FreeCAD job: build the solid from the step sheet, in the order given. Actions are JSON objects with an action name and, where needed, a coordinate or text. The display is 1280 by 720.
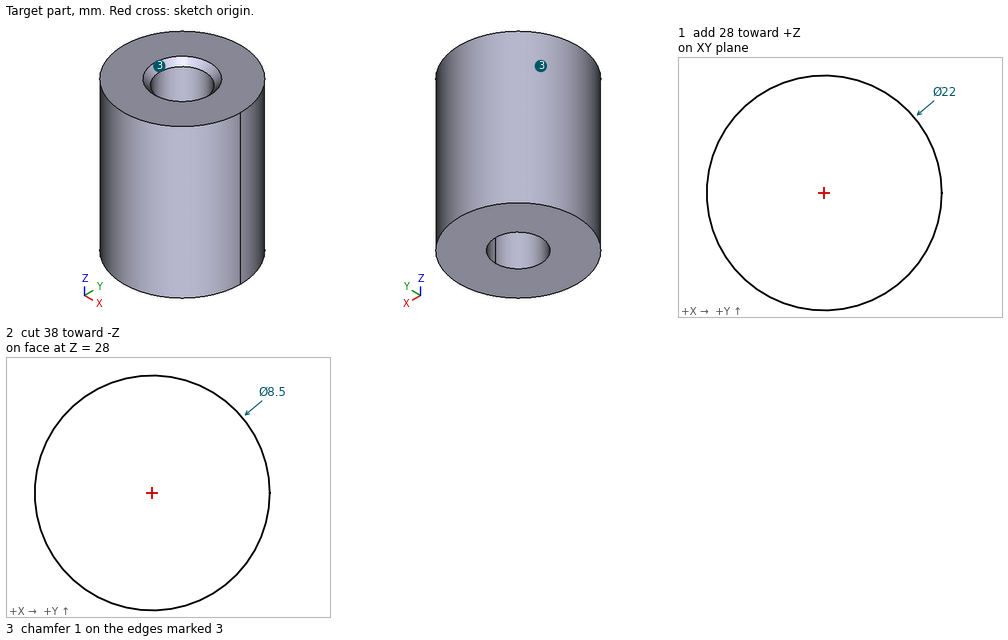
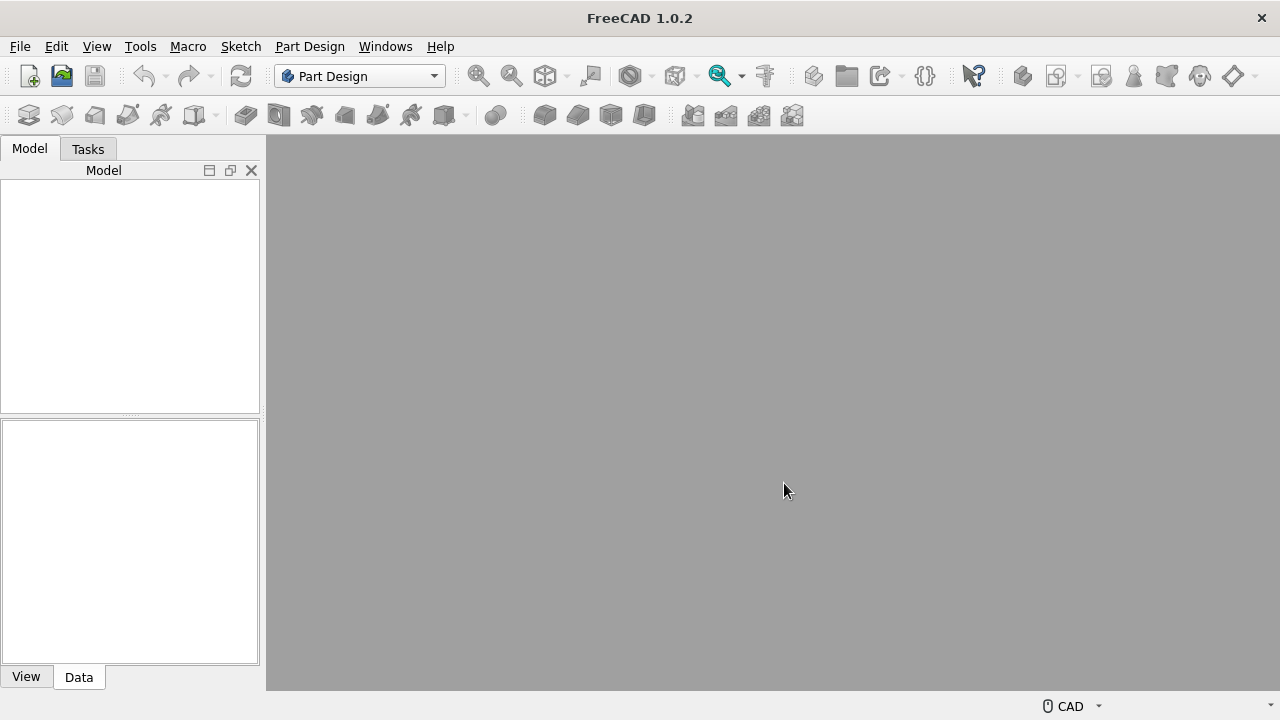
{"action": "left_click", "coordinate": [29, 76]}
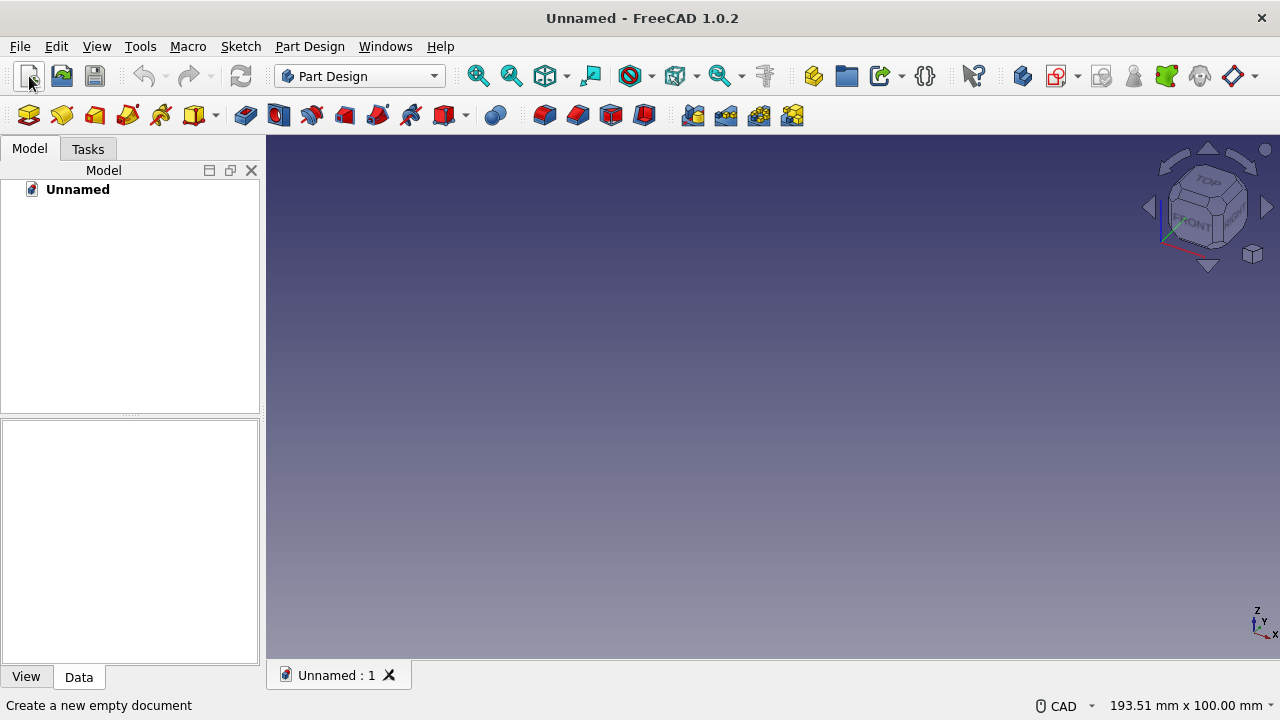
{"action": "left_click", "coordinate": [1056, 76]}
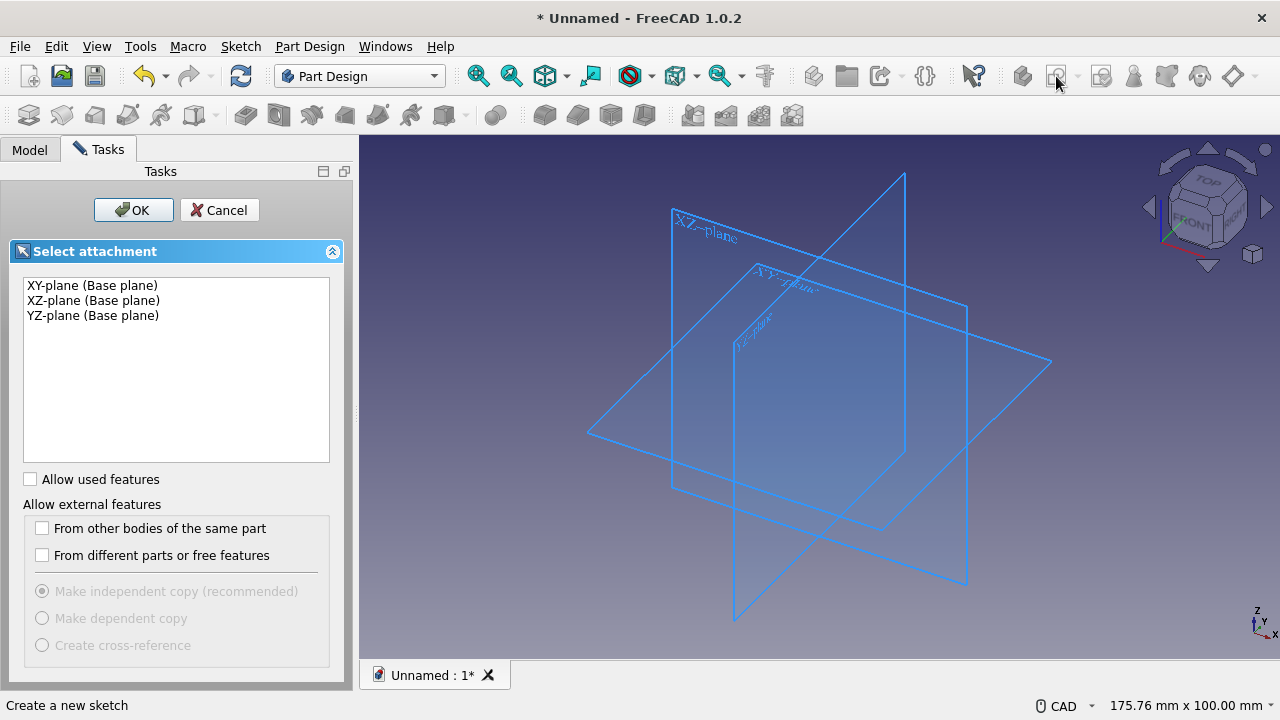
{"action": "left_click", "coordinate": [84, 286]}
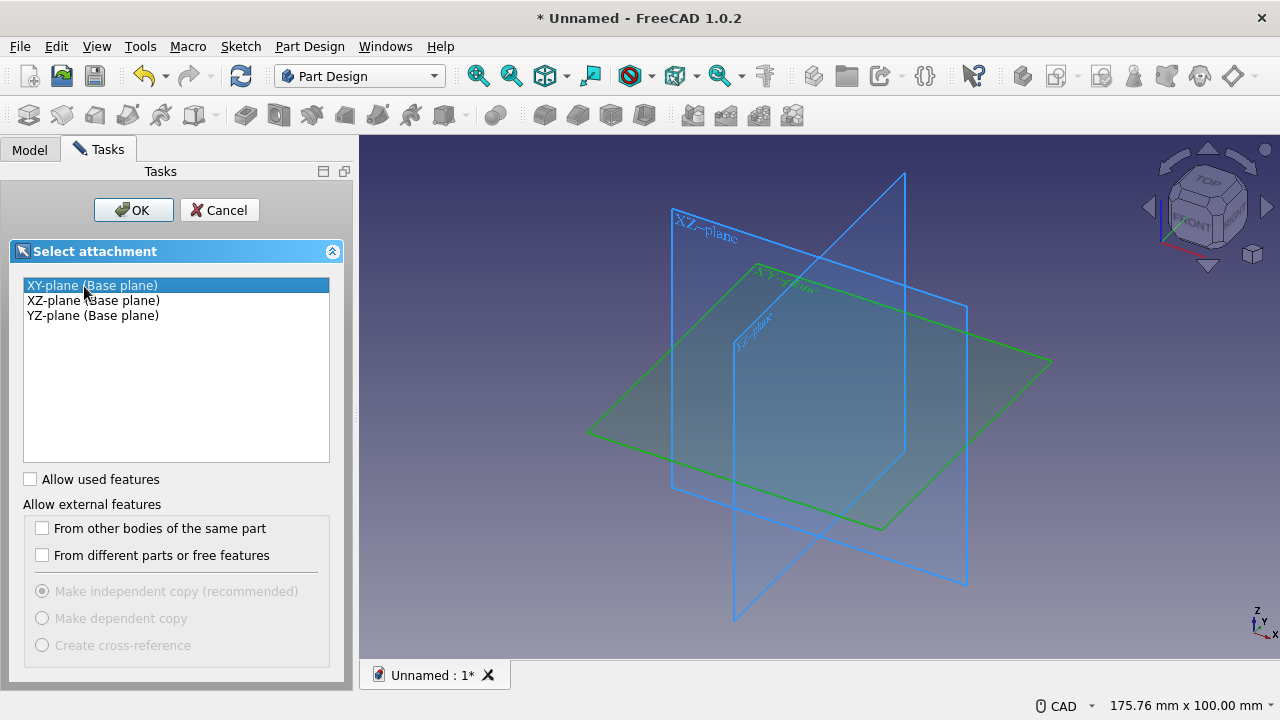
{"action": "left_click", "coordinate": [134, 210]}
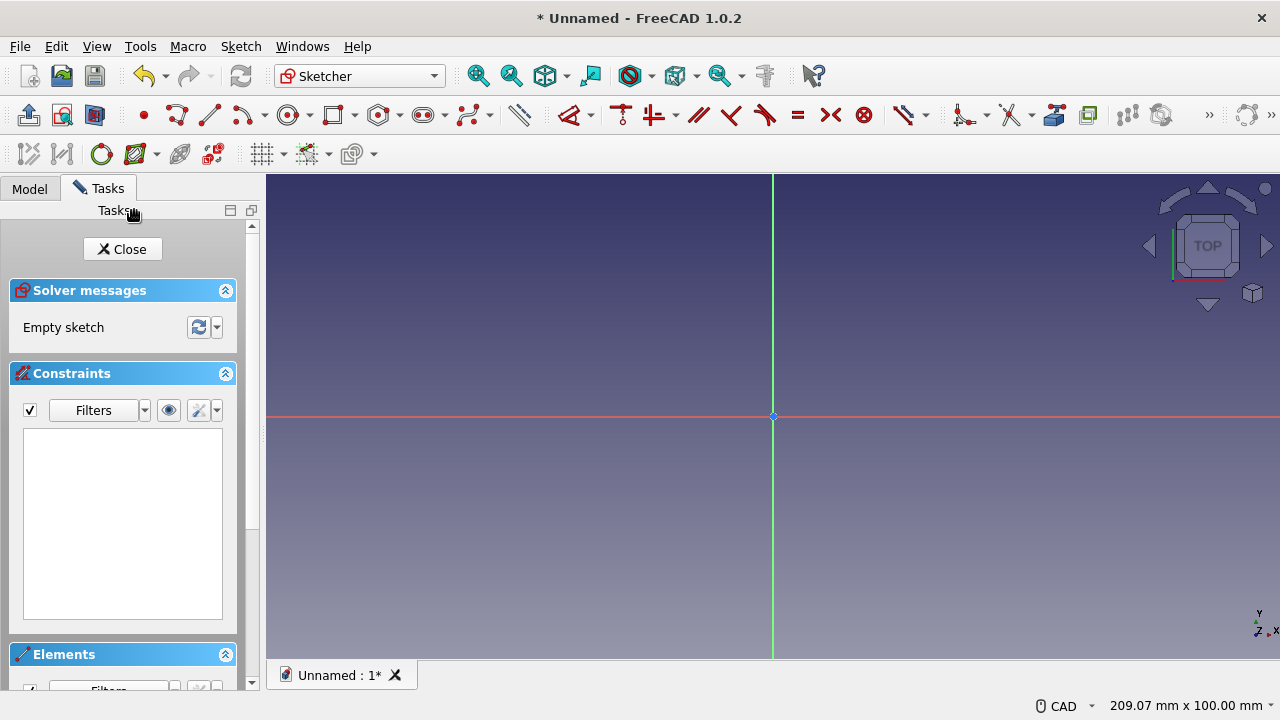
{"action": "scroll", "coordinate": [813, 416], "scroll_direction": "up", "scroll_amount": 5}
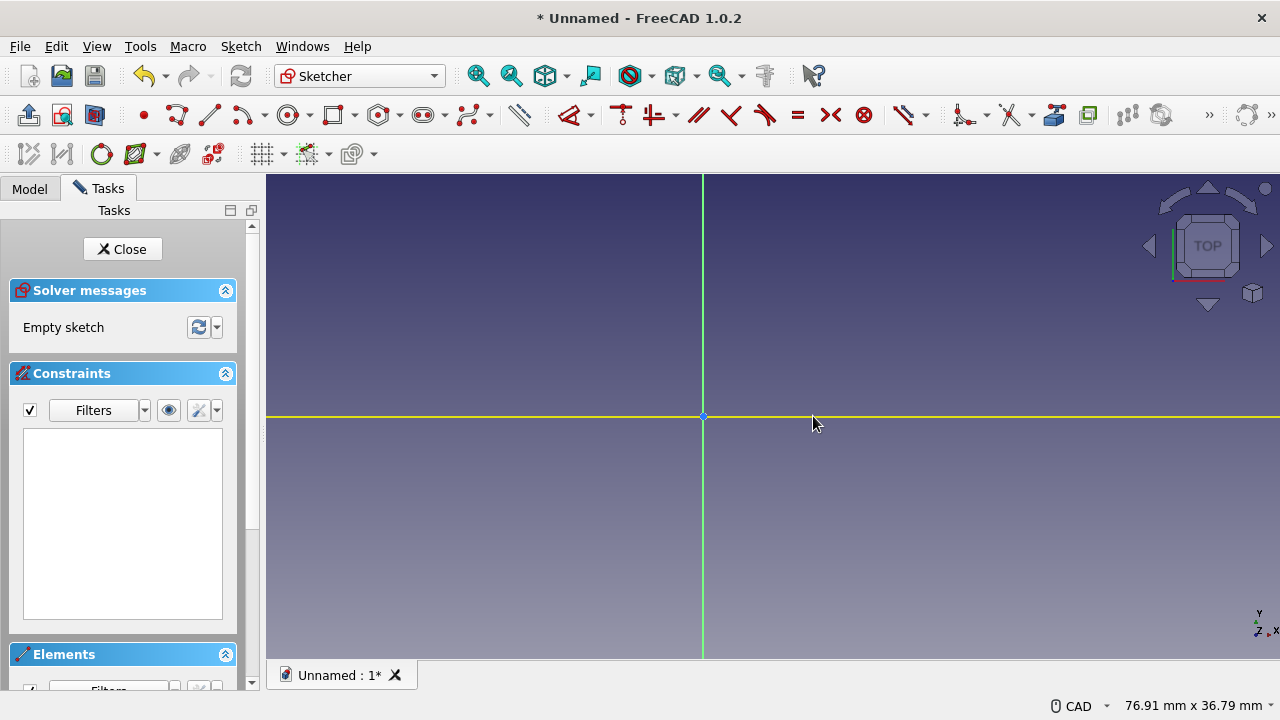
{"action": "left_click", "coordinate": [288, 116]}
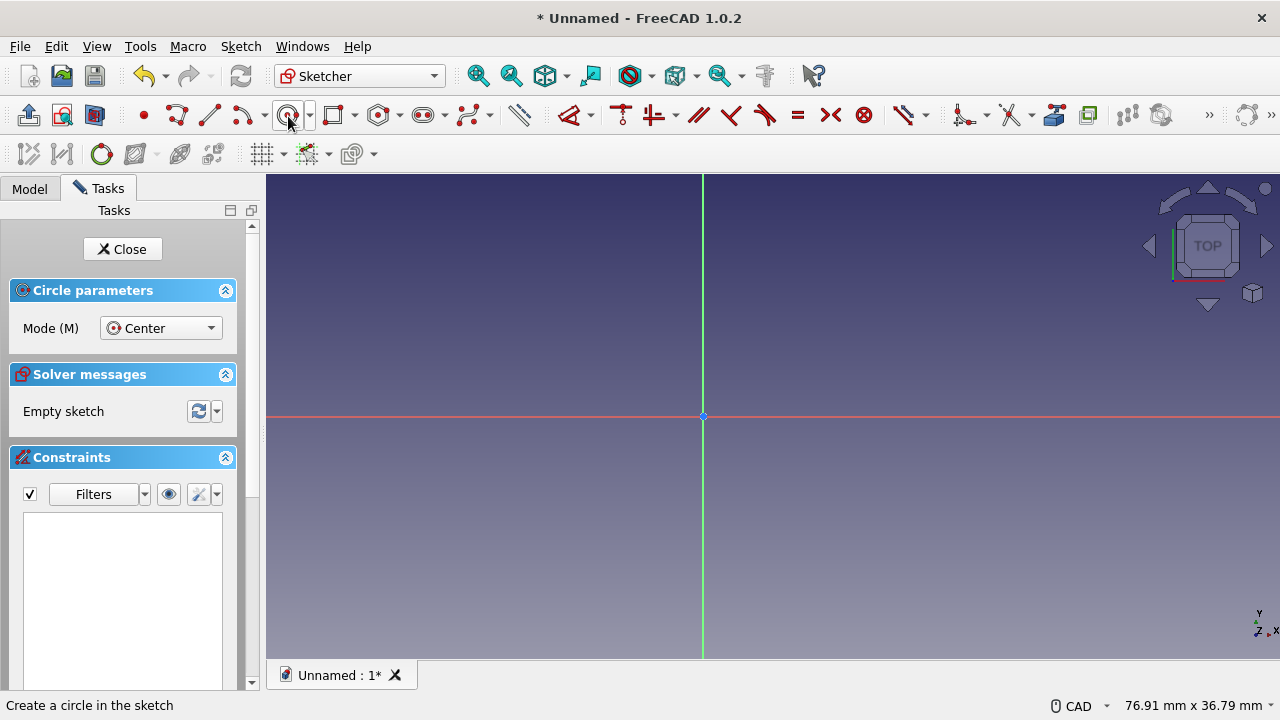
{"action": "left_click", "coordinate": [703, 416]}
{"action": "left_click", "coordinate": [806, 314]}
{"action": "key", "text": "Escape"}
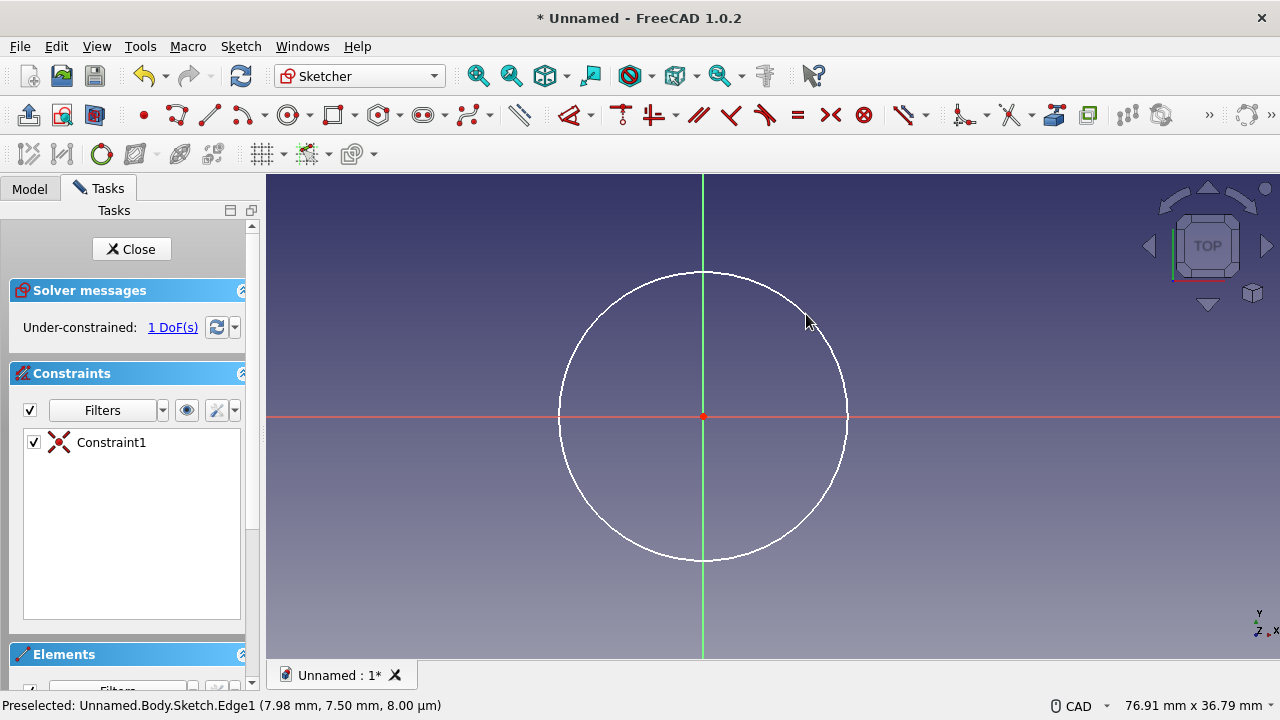
{"action": "left_click", "coordinate": [805, 314]}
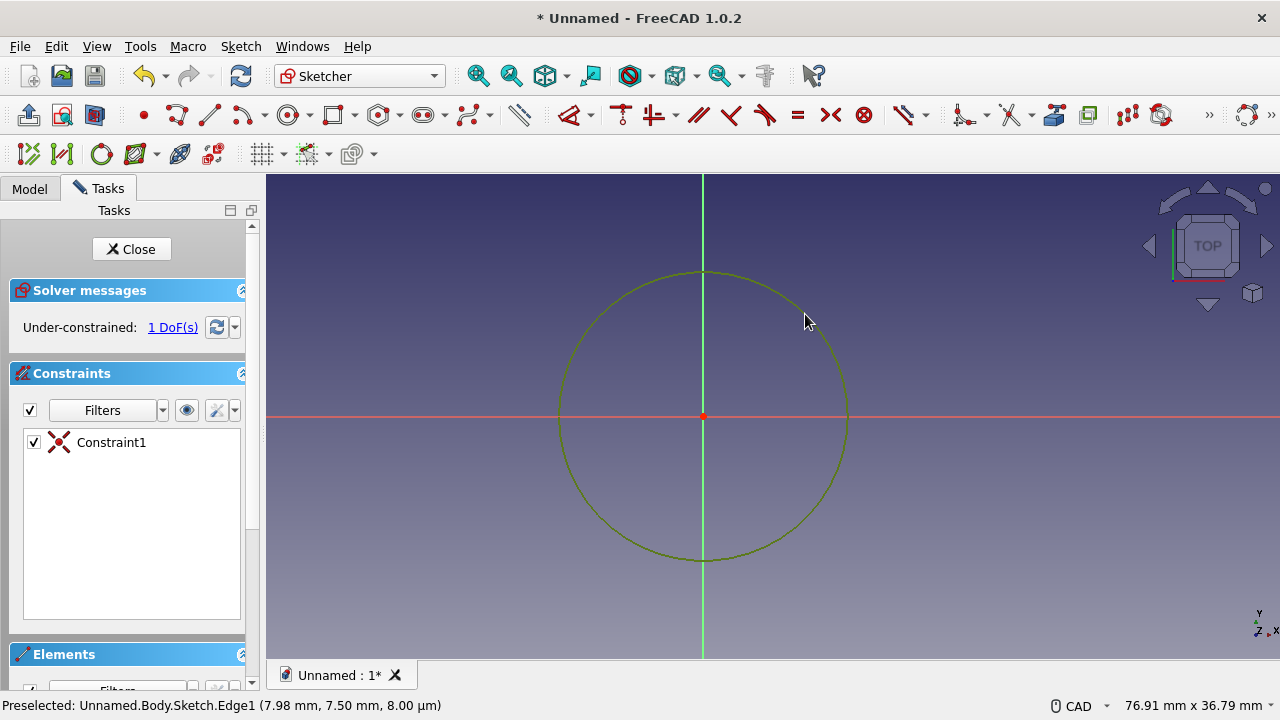
{"action": "left_click", "coordinate": [590, 116]}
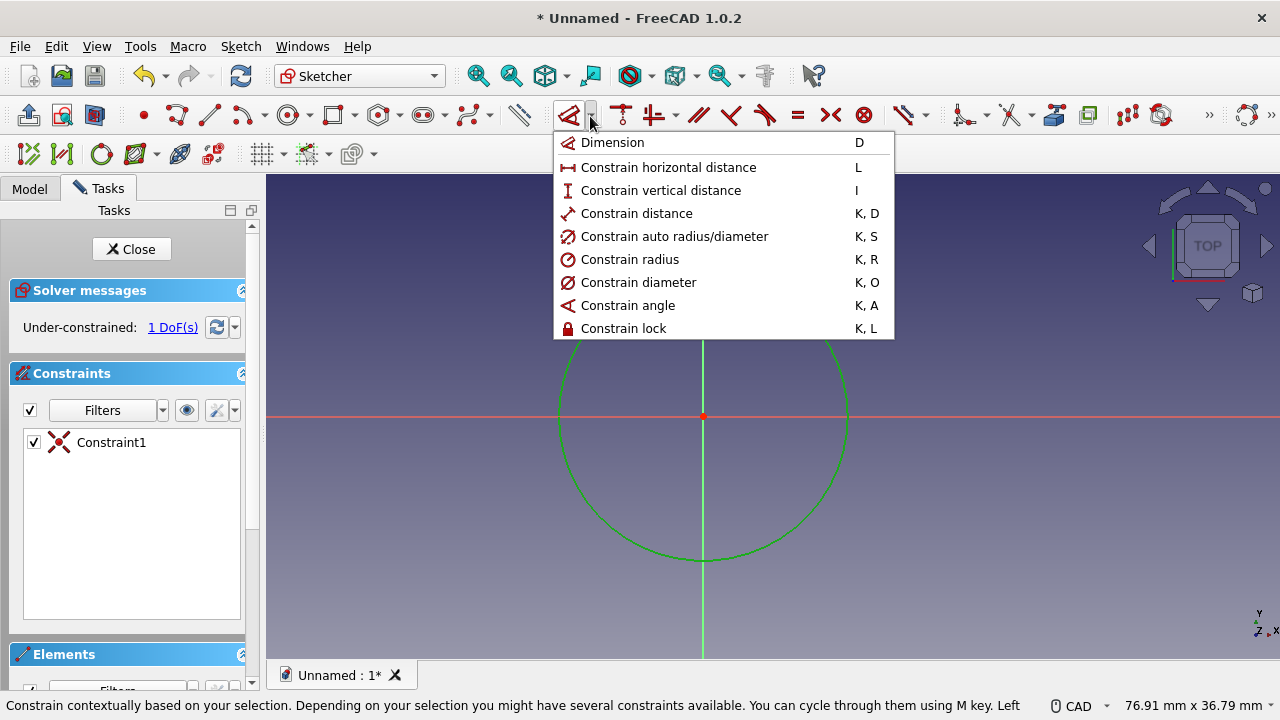
{"action": "left_click", "coordinate": [724, 282]}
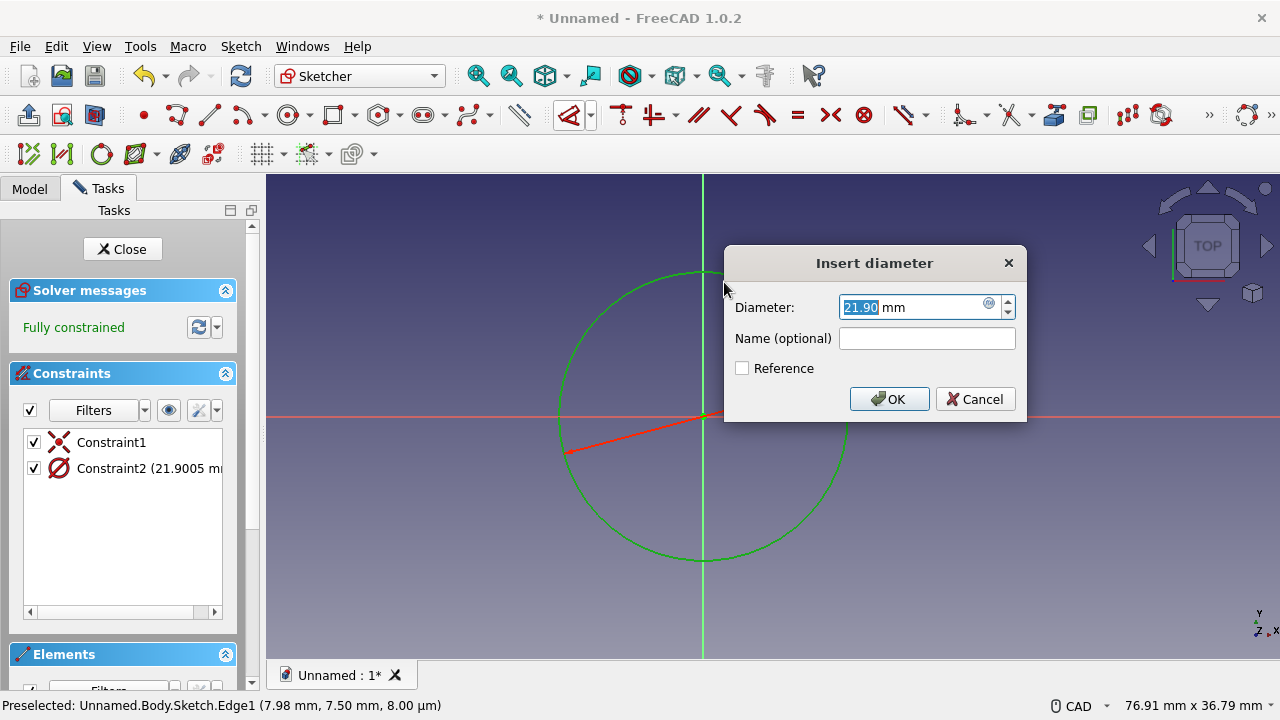
{"action": "type", "text": "22"}
{"action": "key", "text": "Return"}